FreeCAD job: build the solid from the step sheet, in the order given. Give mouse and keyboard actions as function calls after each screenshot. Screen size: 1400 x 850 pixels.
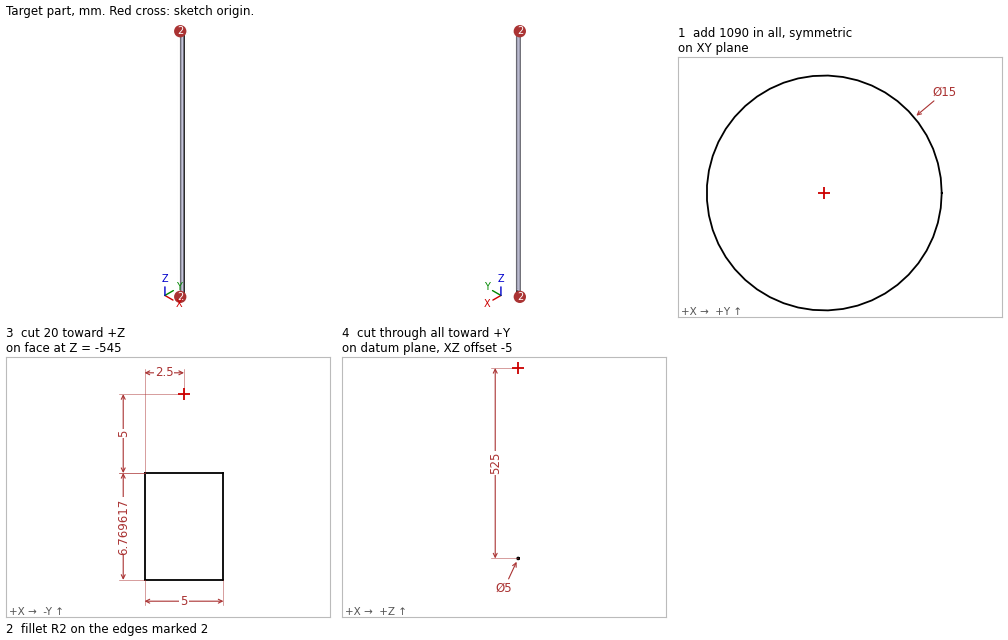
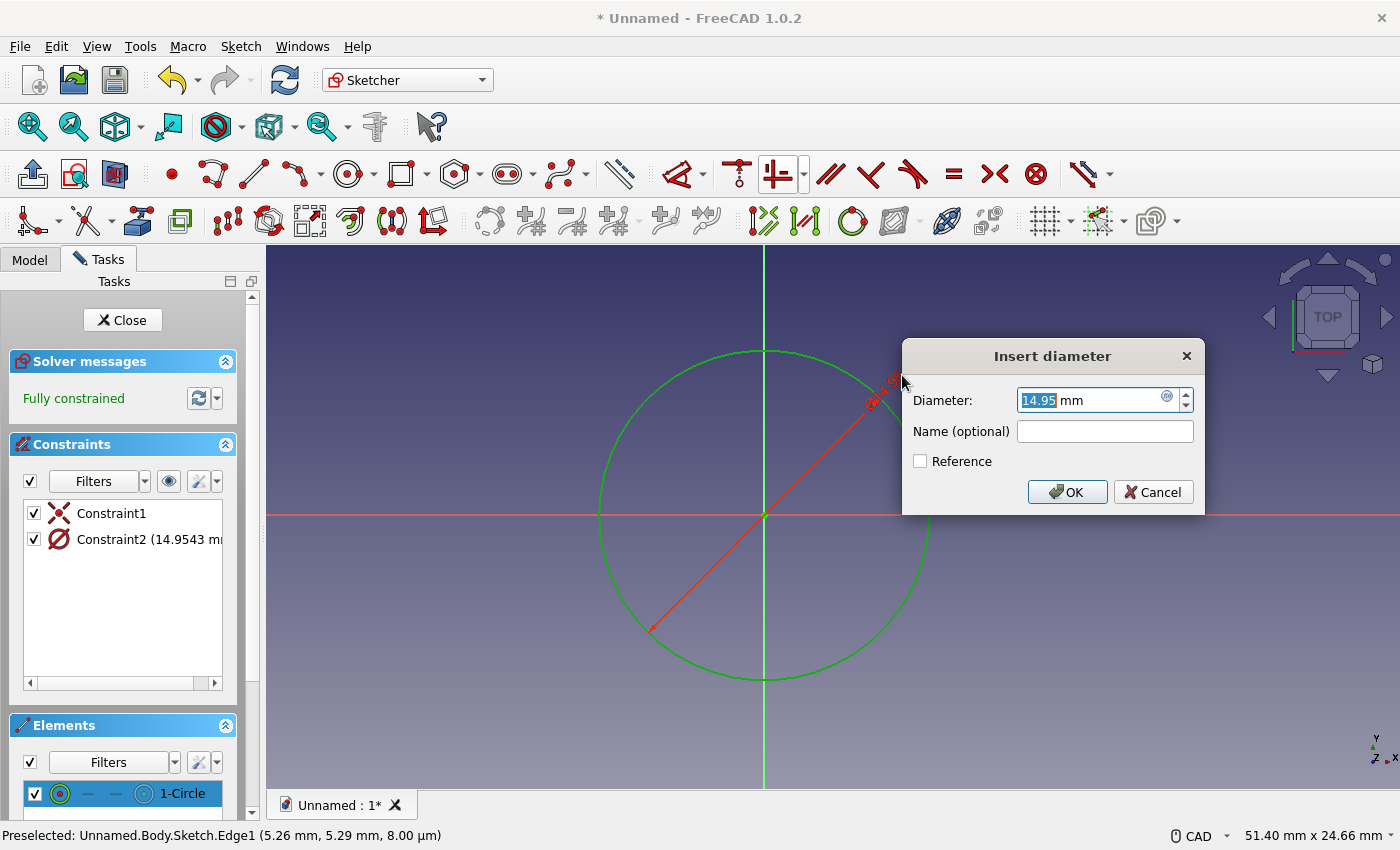
text(15)
key(Return)
key(Escape)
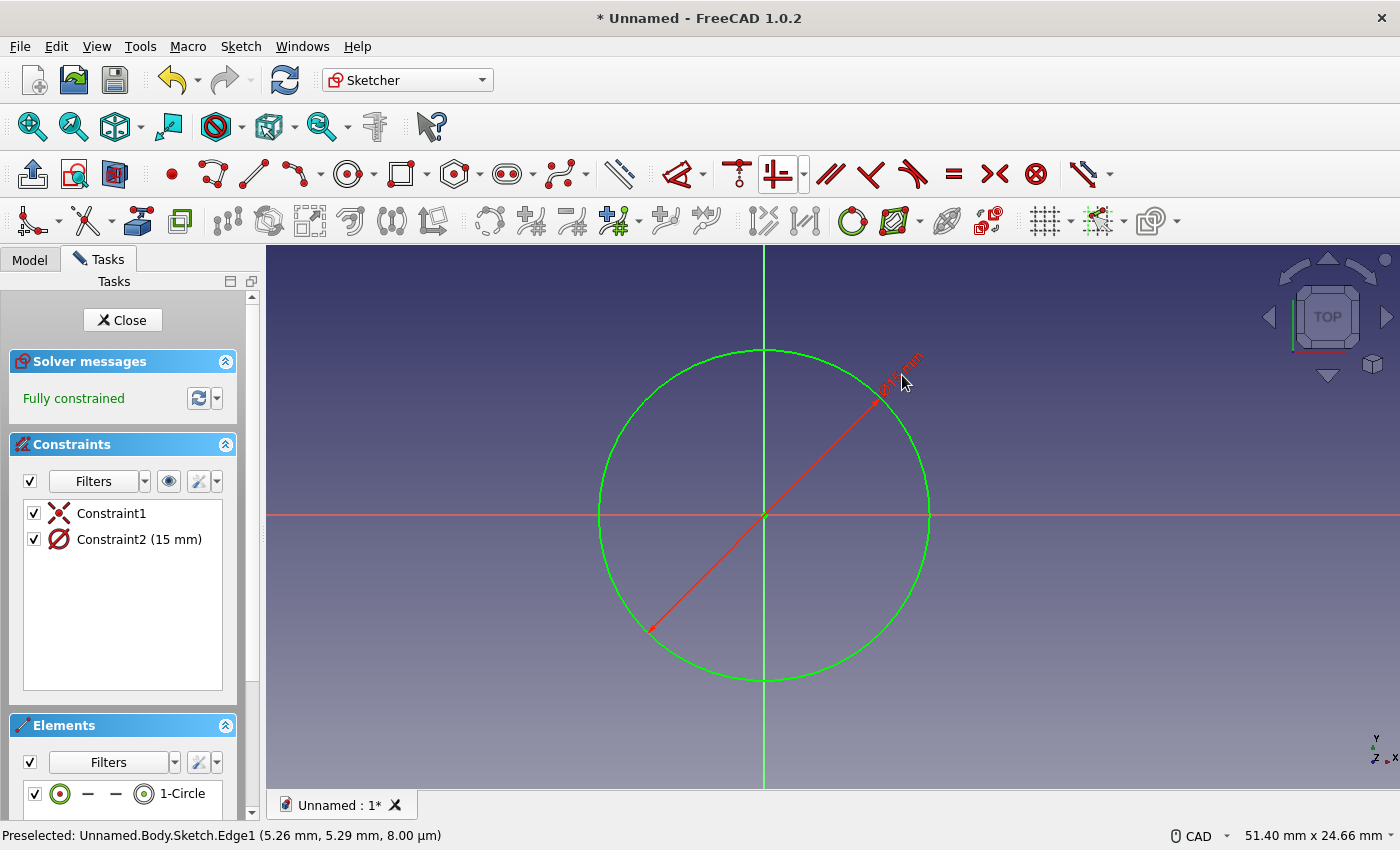
click(123, 320)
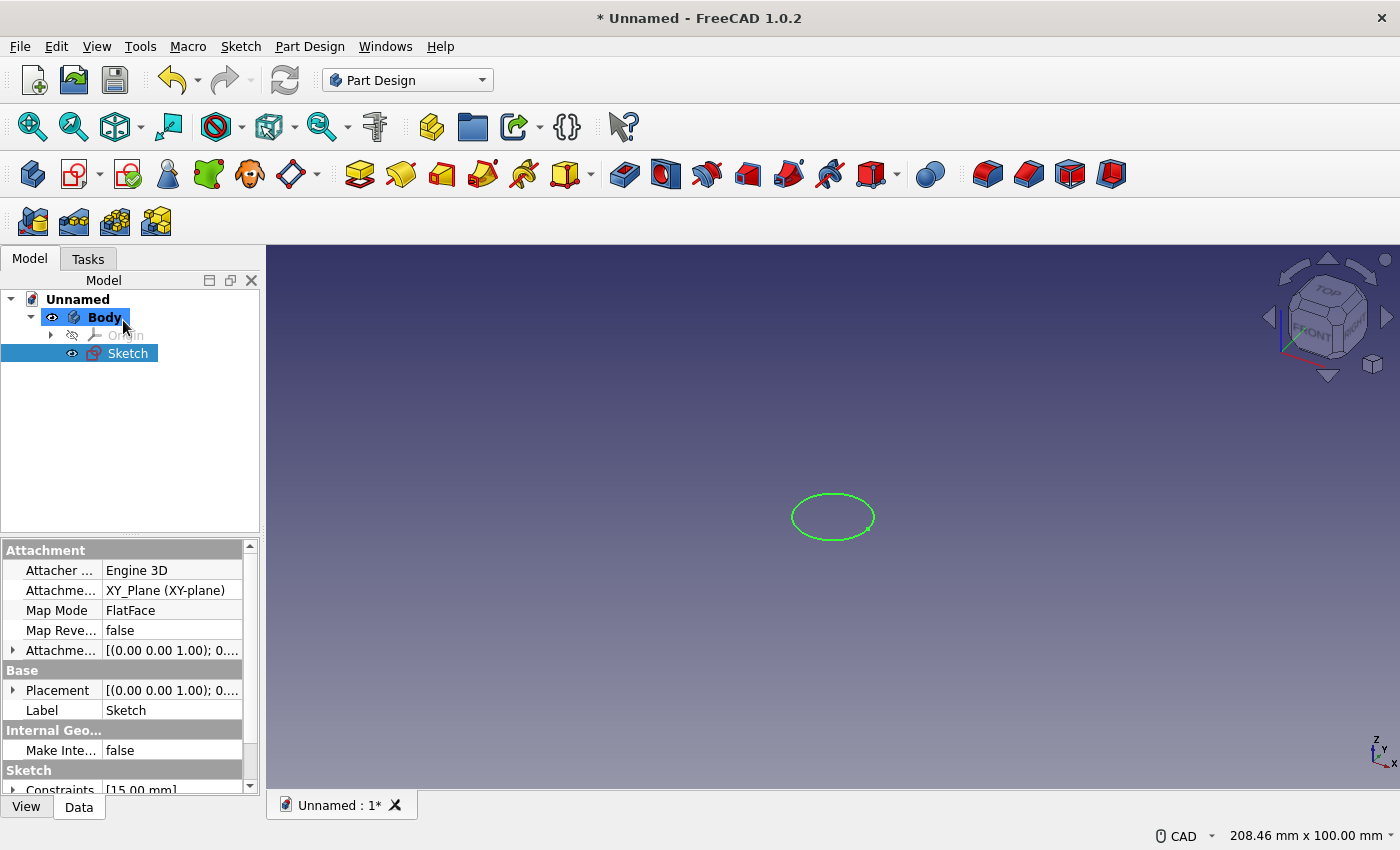
click(360, 174)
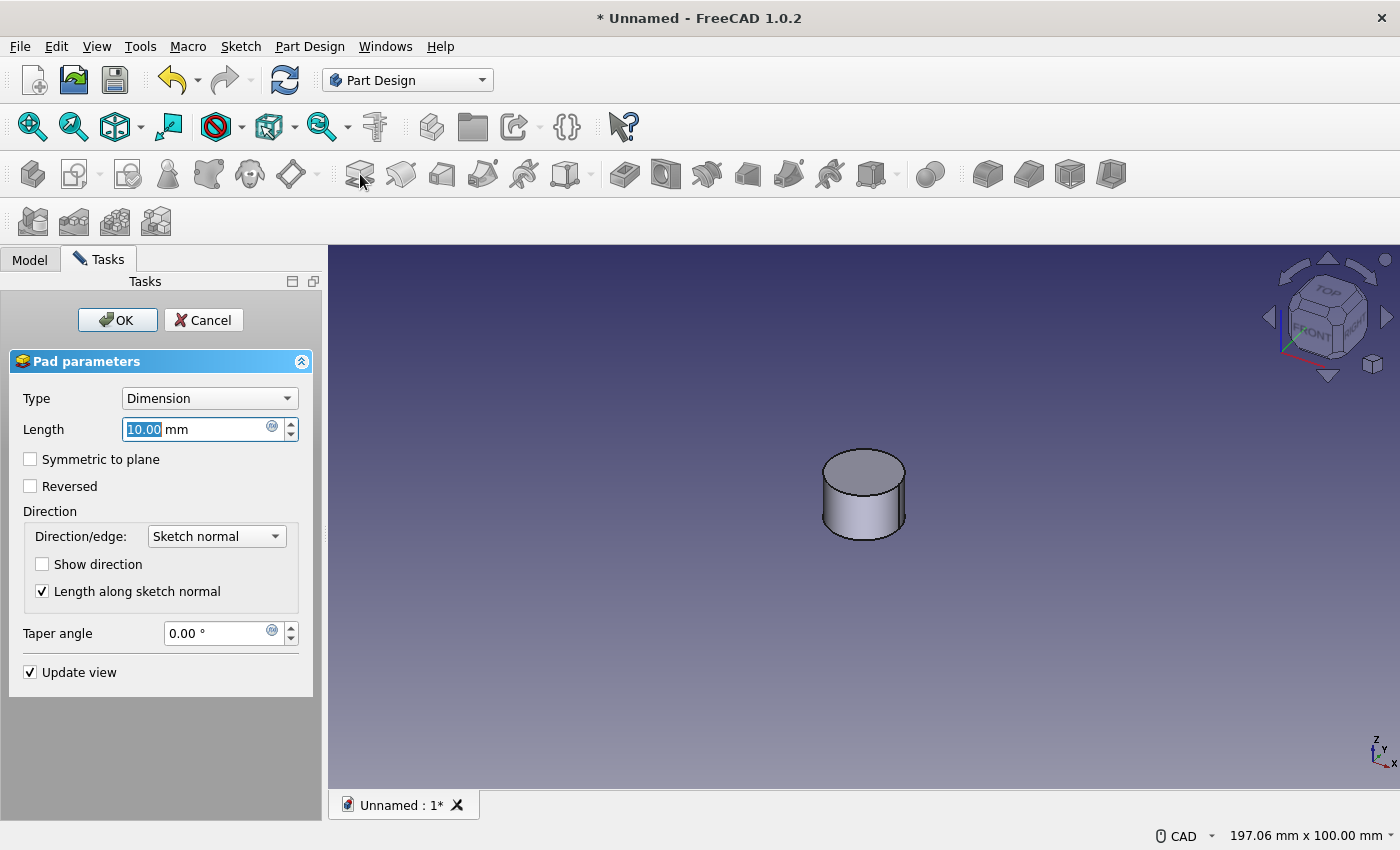
text(1090)
key(Tab)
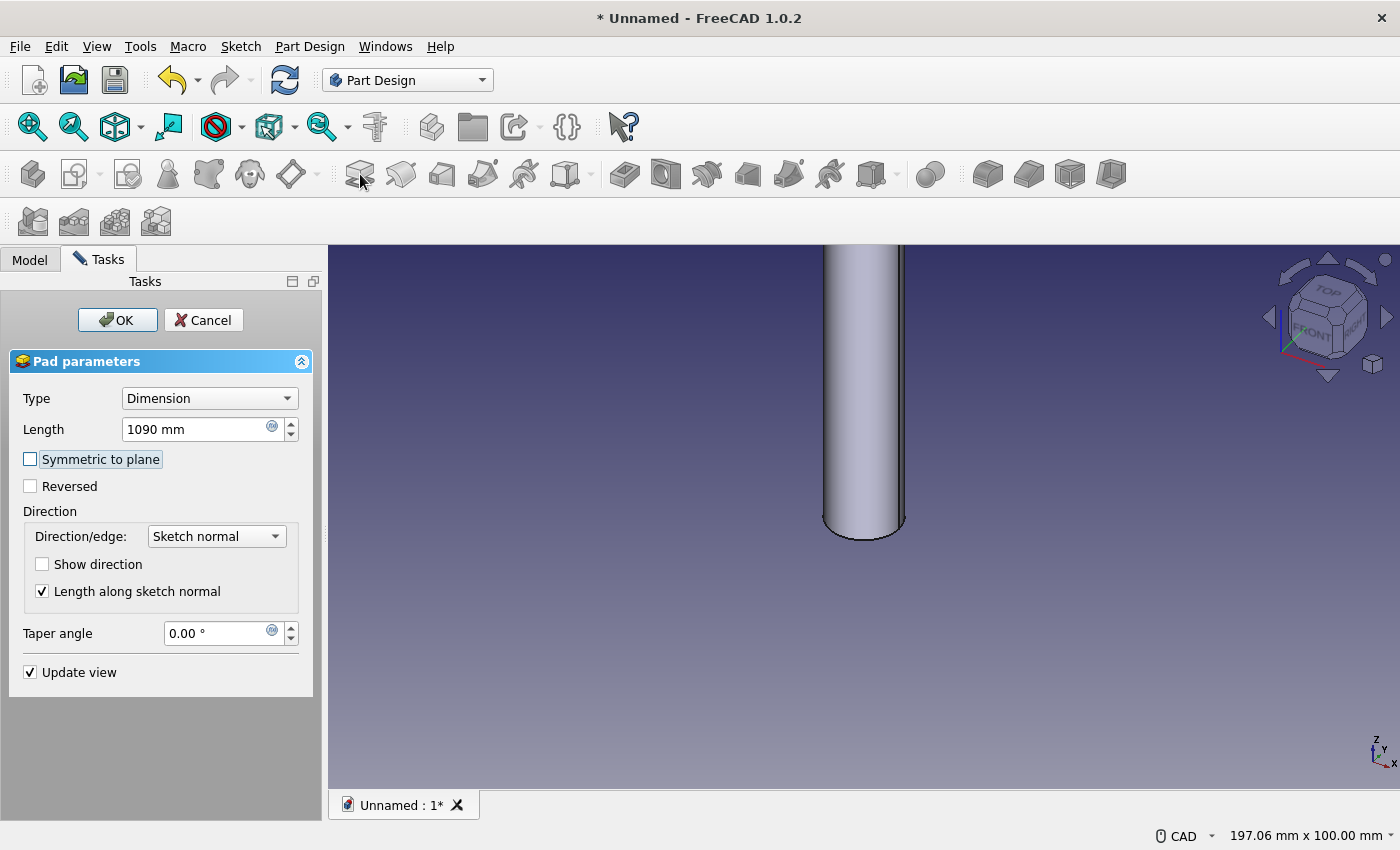
click(31, 459)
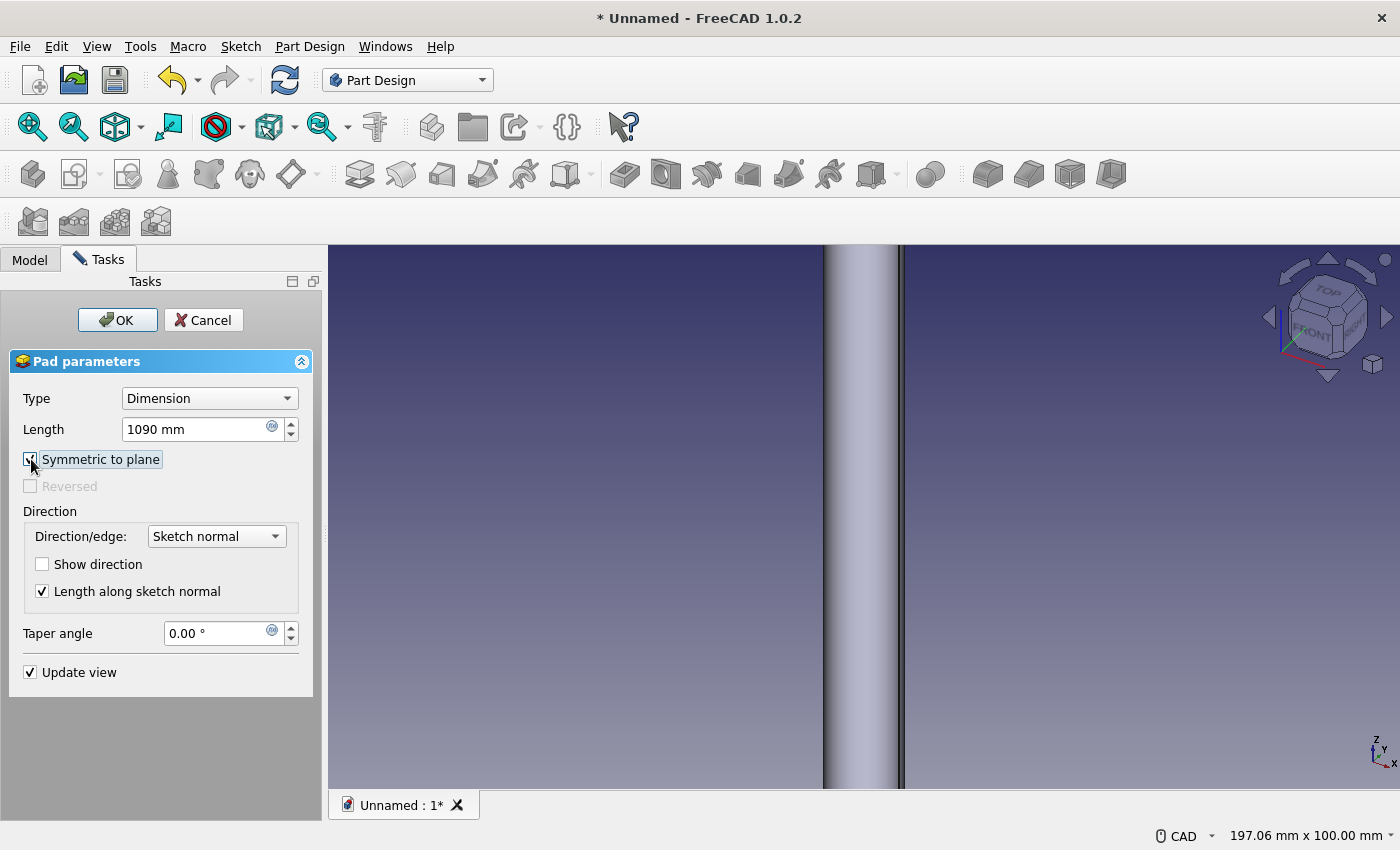
click(118, 320)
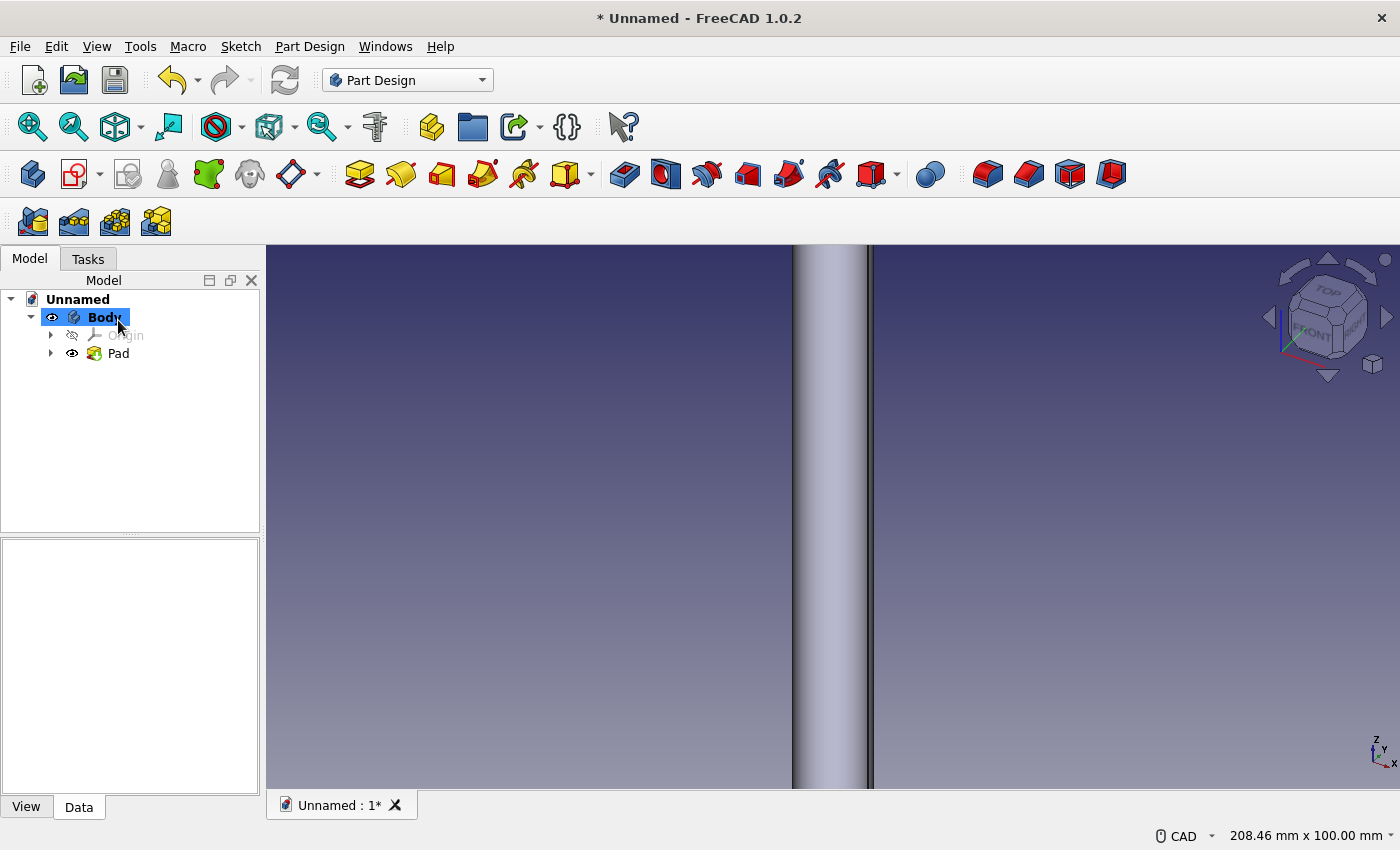
key(v)
key(f)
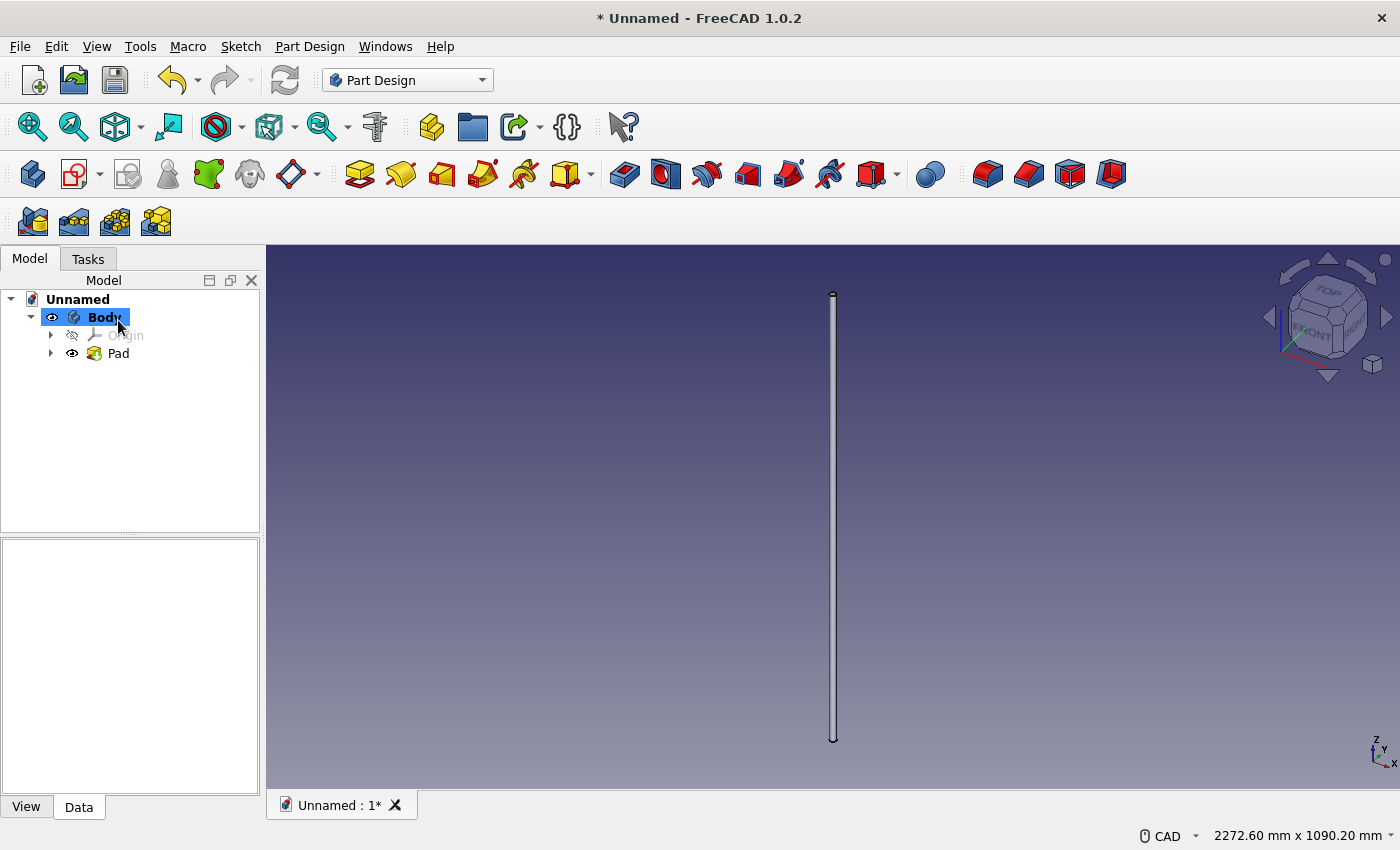
click(830, 292)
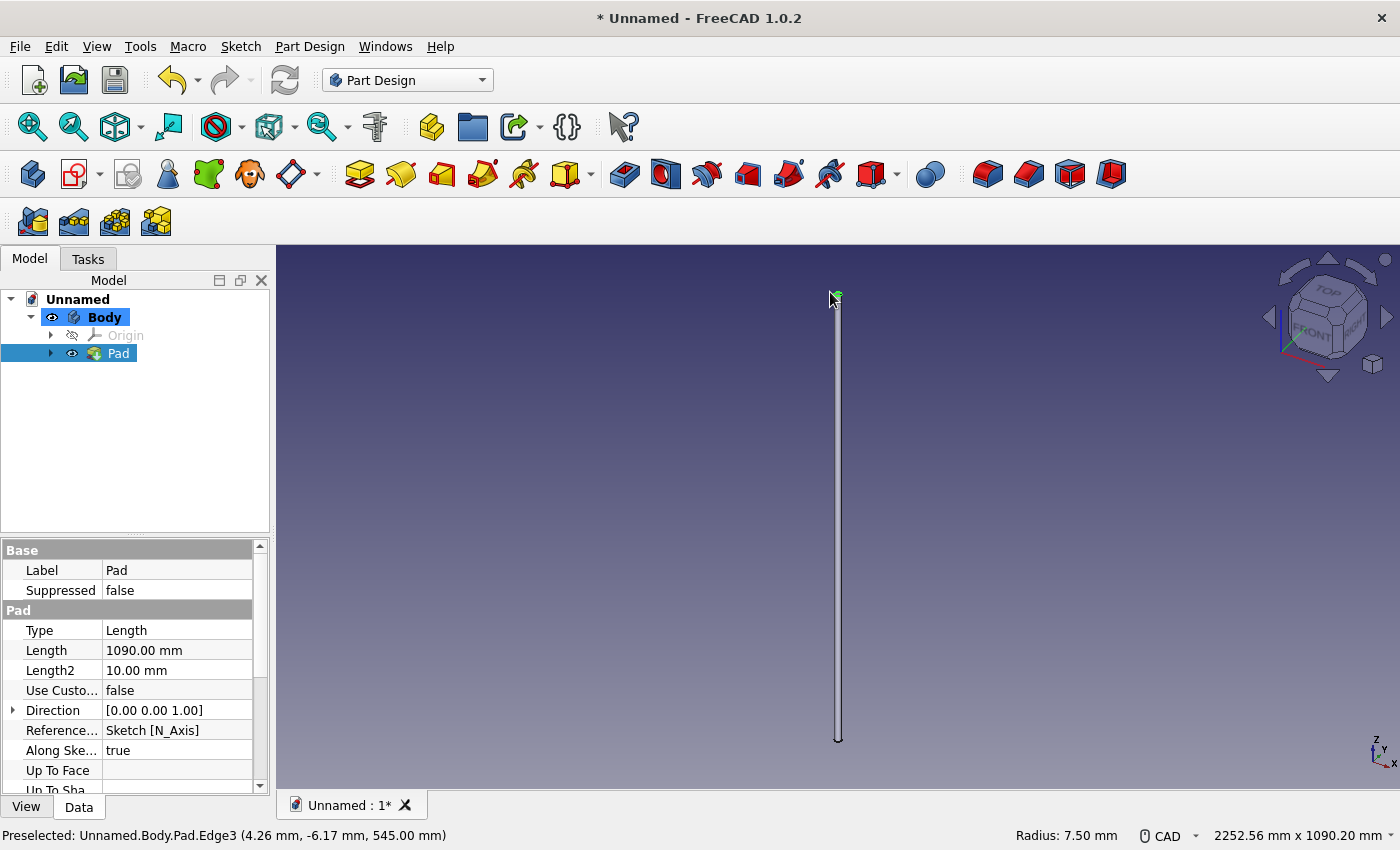
key(0)